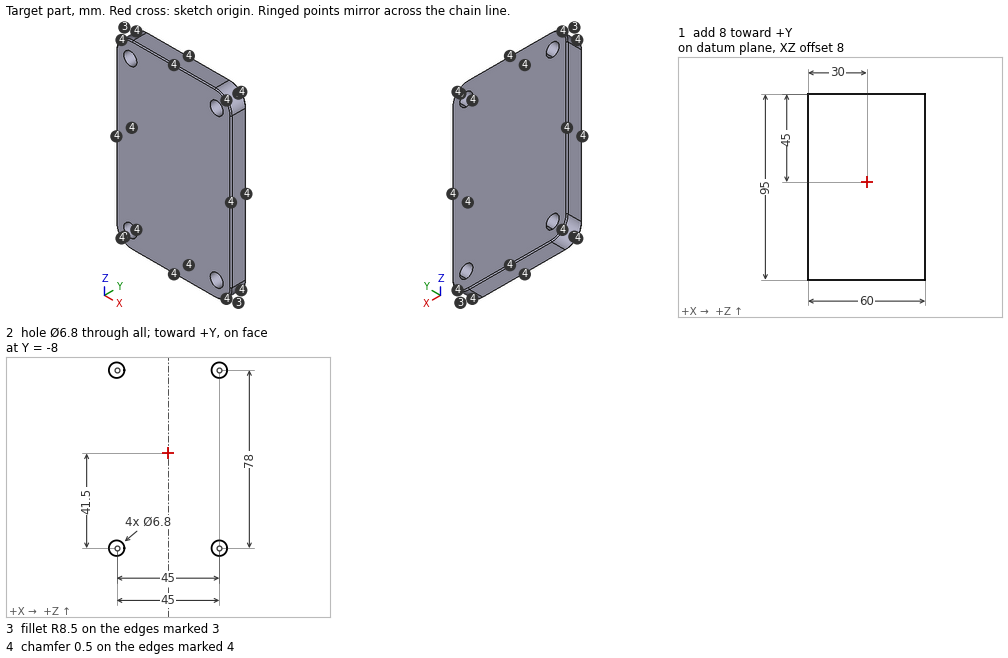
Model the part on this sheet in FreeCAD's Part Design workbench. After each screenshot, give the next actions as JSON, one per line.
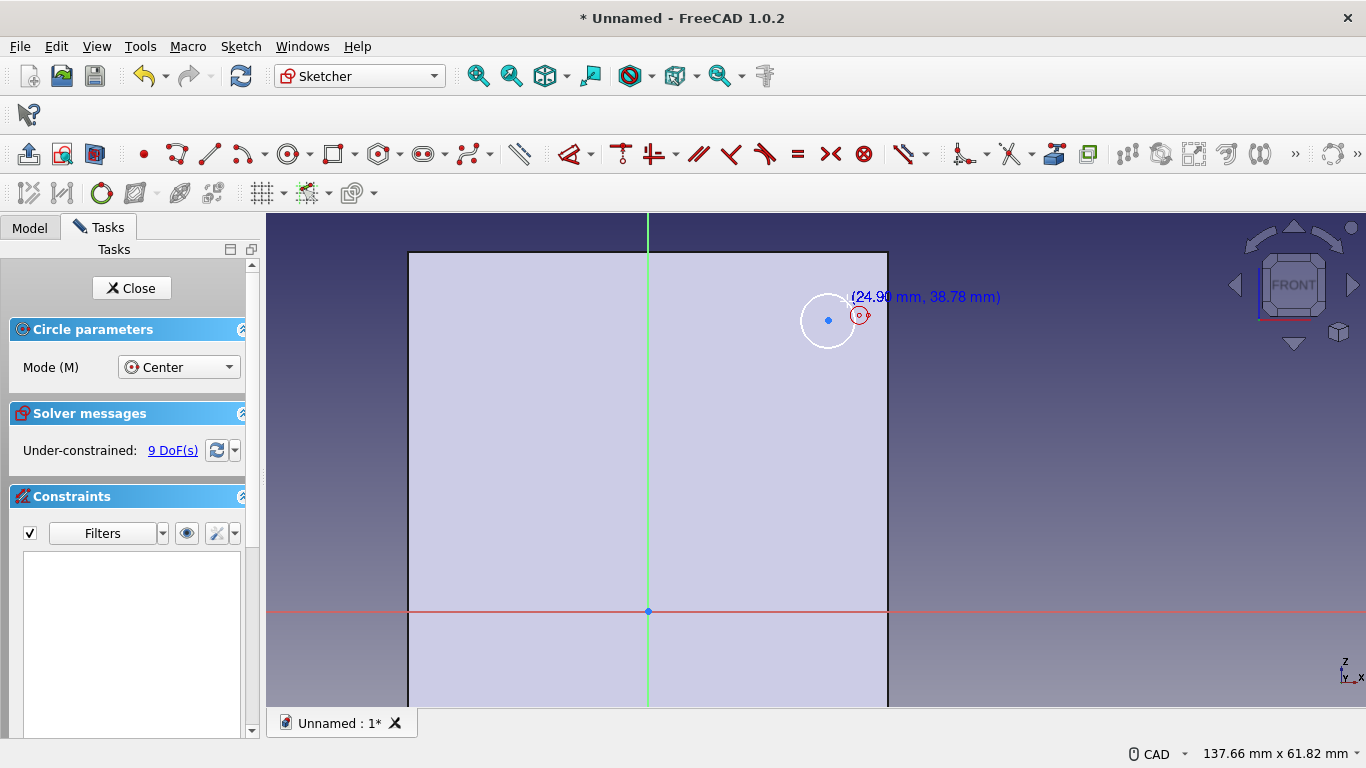
{"action": "left_click", "coordinate": [468, 320]}
{"action": "left_click", "coordinate": [487, 301]}
{"action": "key", "text": "Escape"}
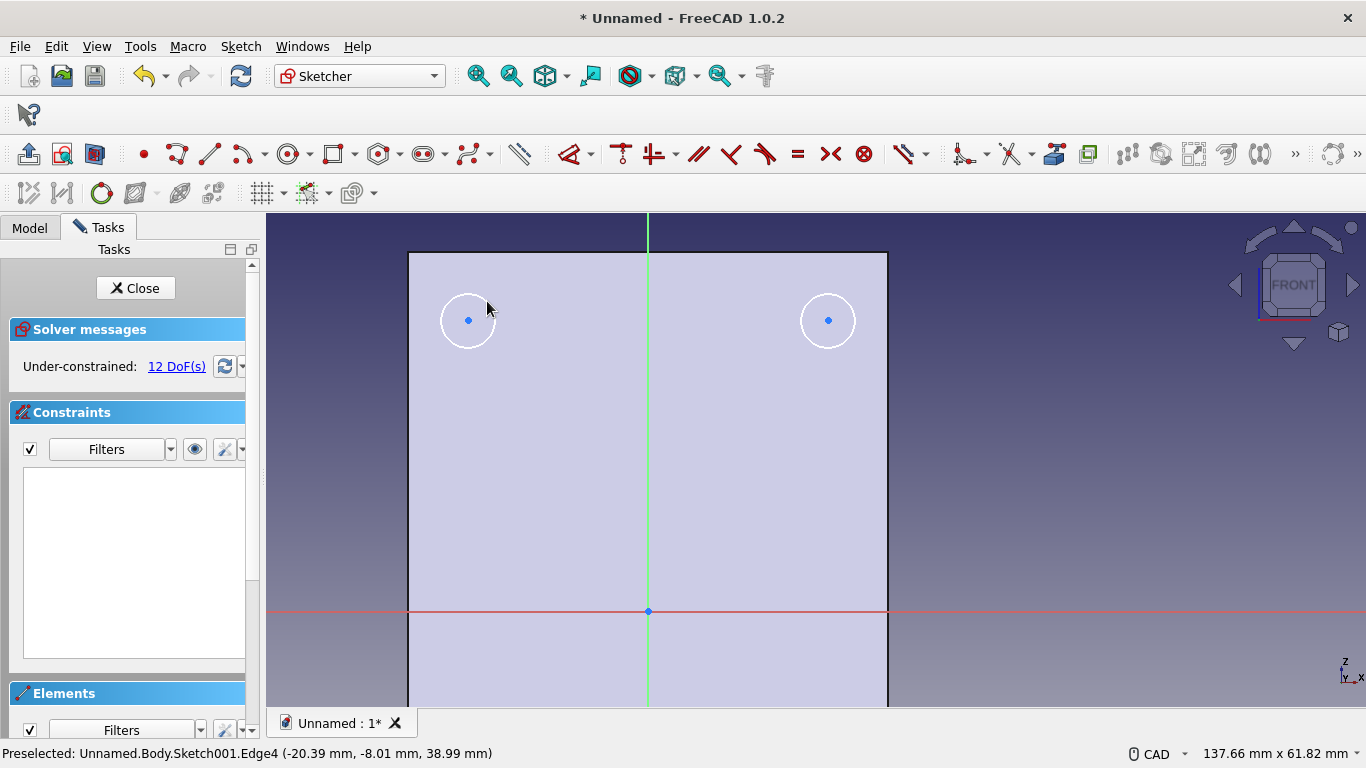
{"action": "scroll", "coordinate": [829, 320], "scroll_direction": "down", "scroll_amount": 4}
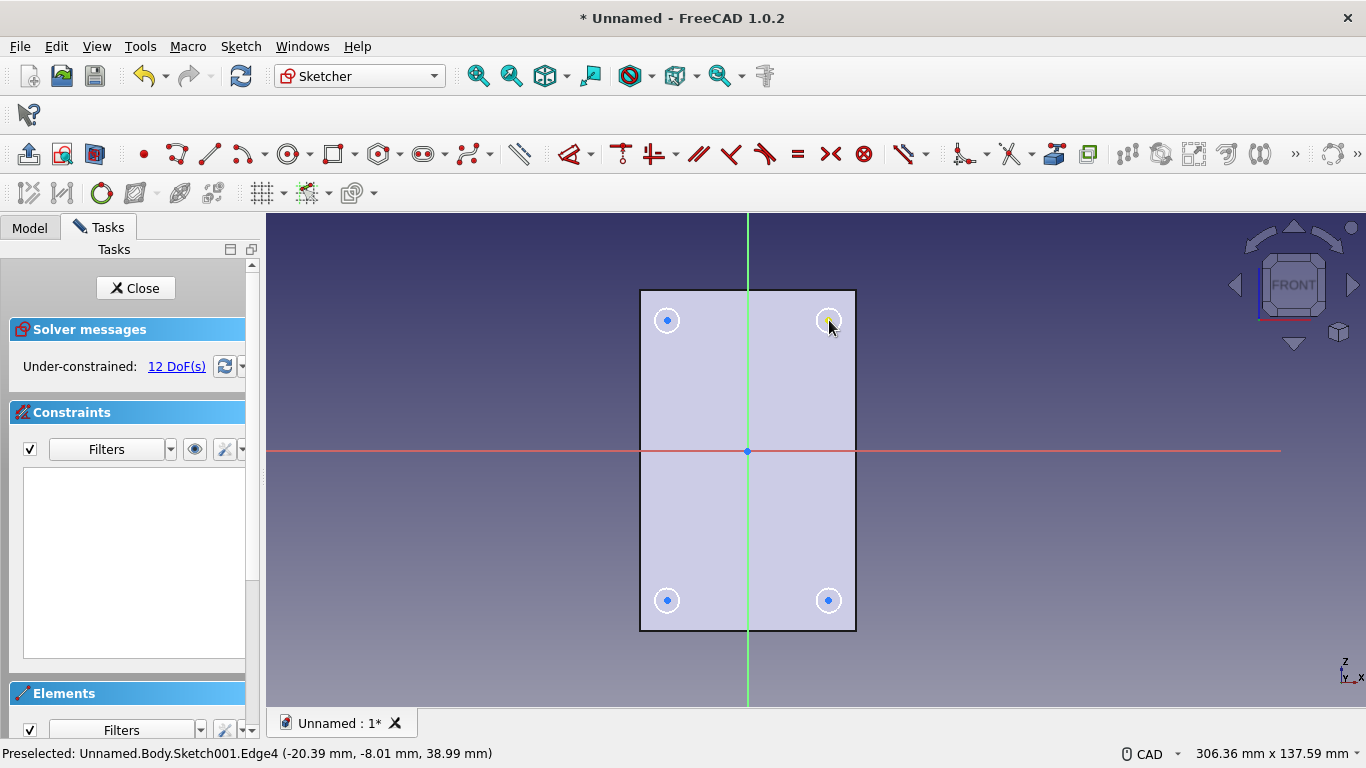
{"action": "left_click", "coordinate": [676, 592]}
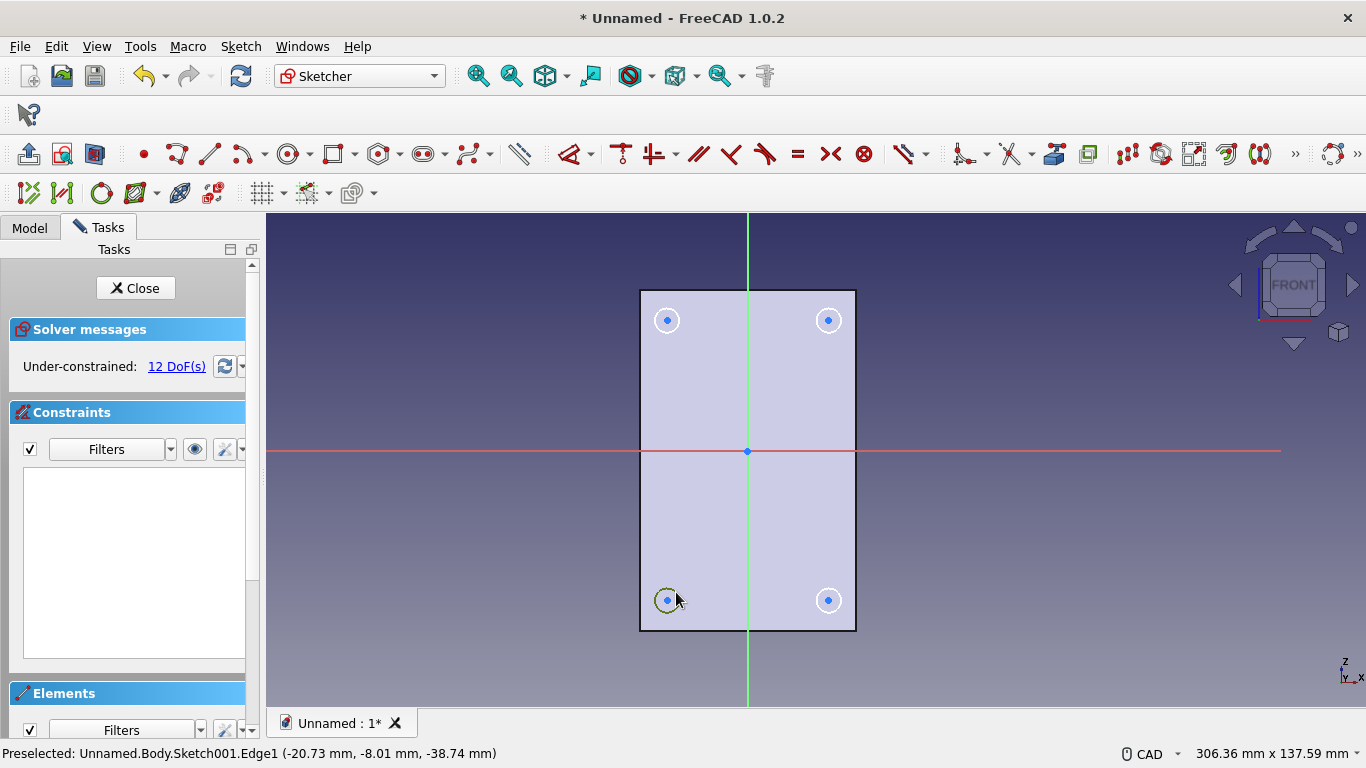
{"action": "left_click", "coordinate": [837, 592]}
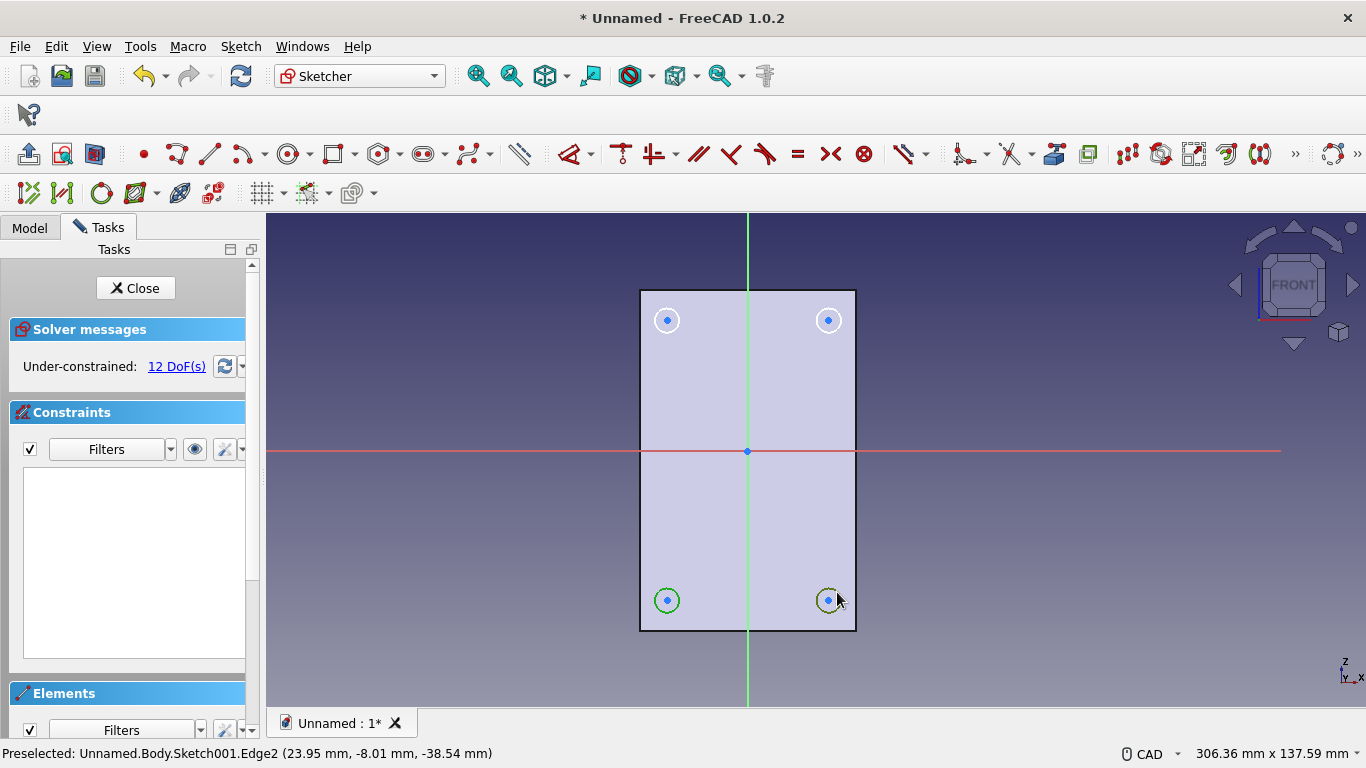
{"action": "left_click", "coordinate": [837, 312]}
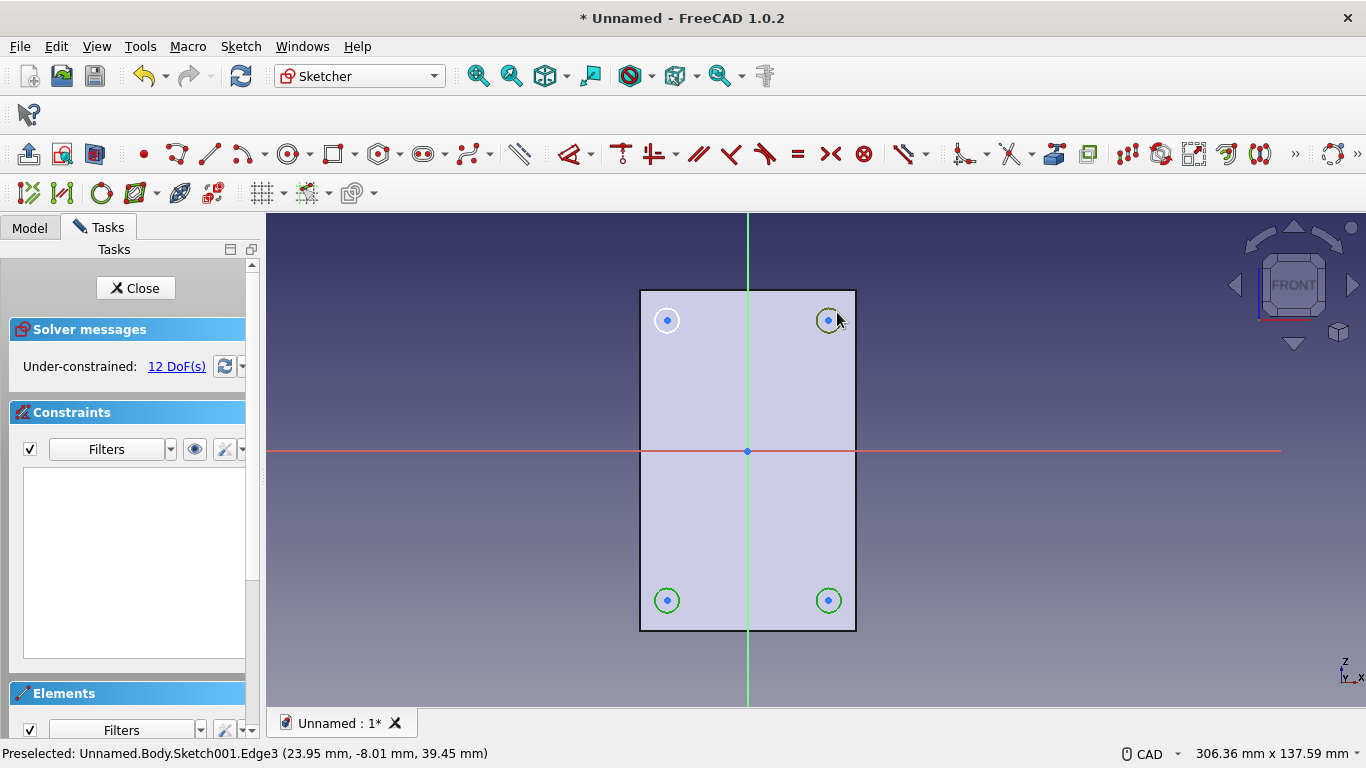
{"action": "left_click", "coordinate": [676, 312]}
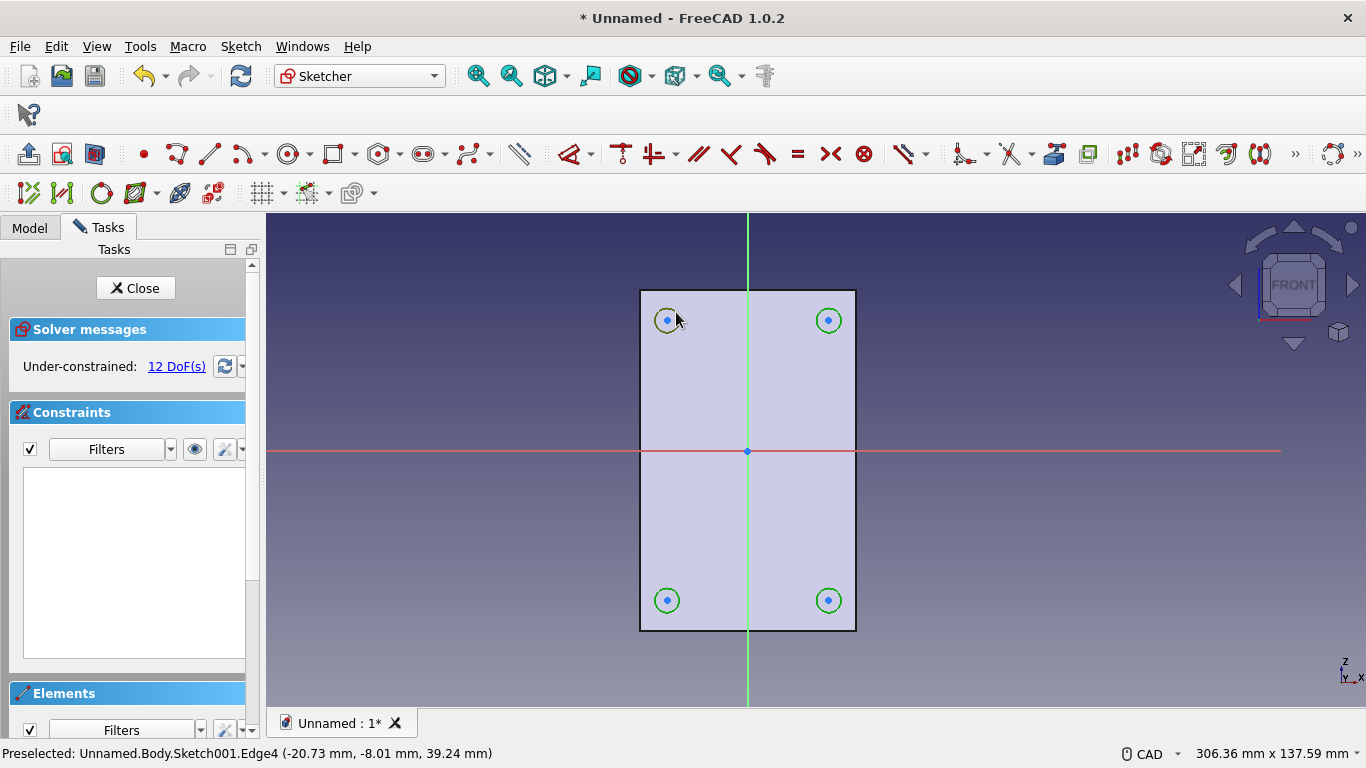
{"action": "left_click", "coordinate": [798, 154]}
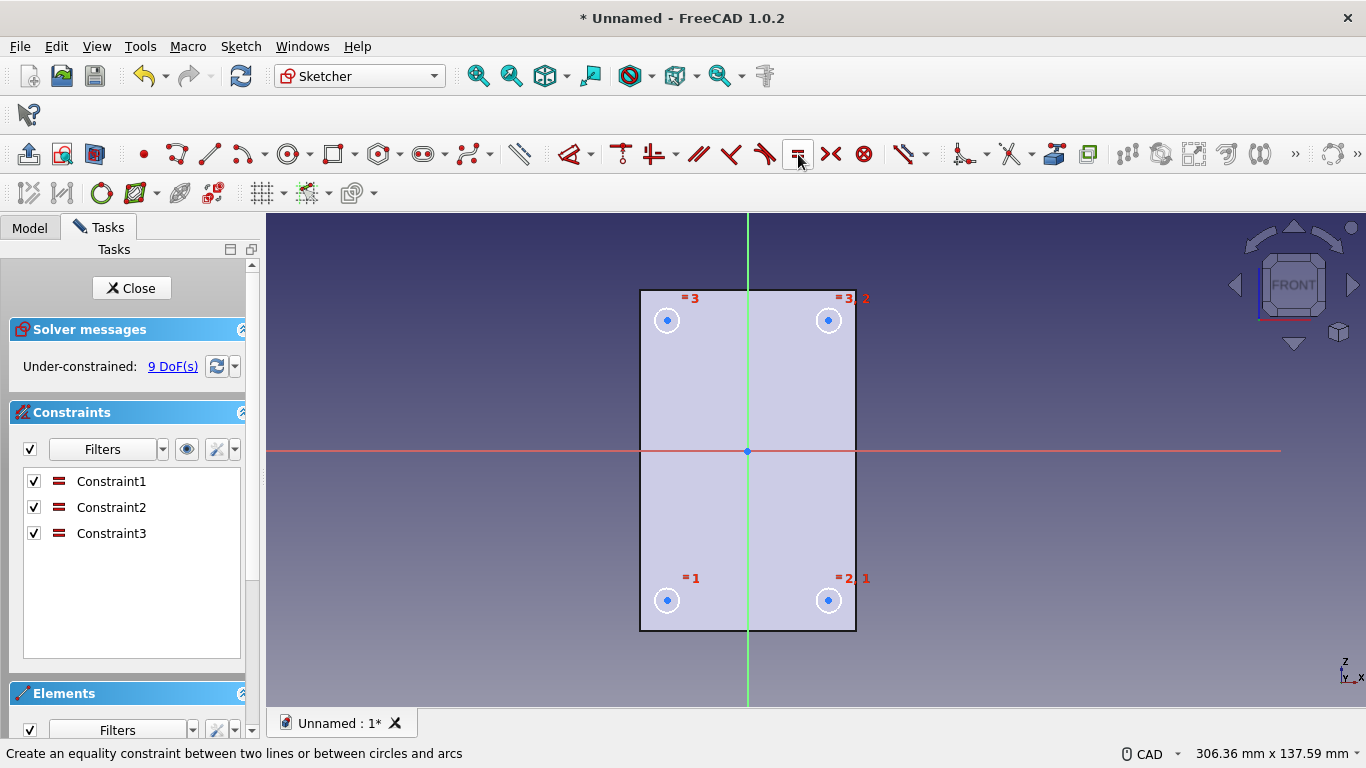
{"action": "left_click", "coordinate": [667, 601]}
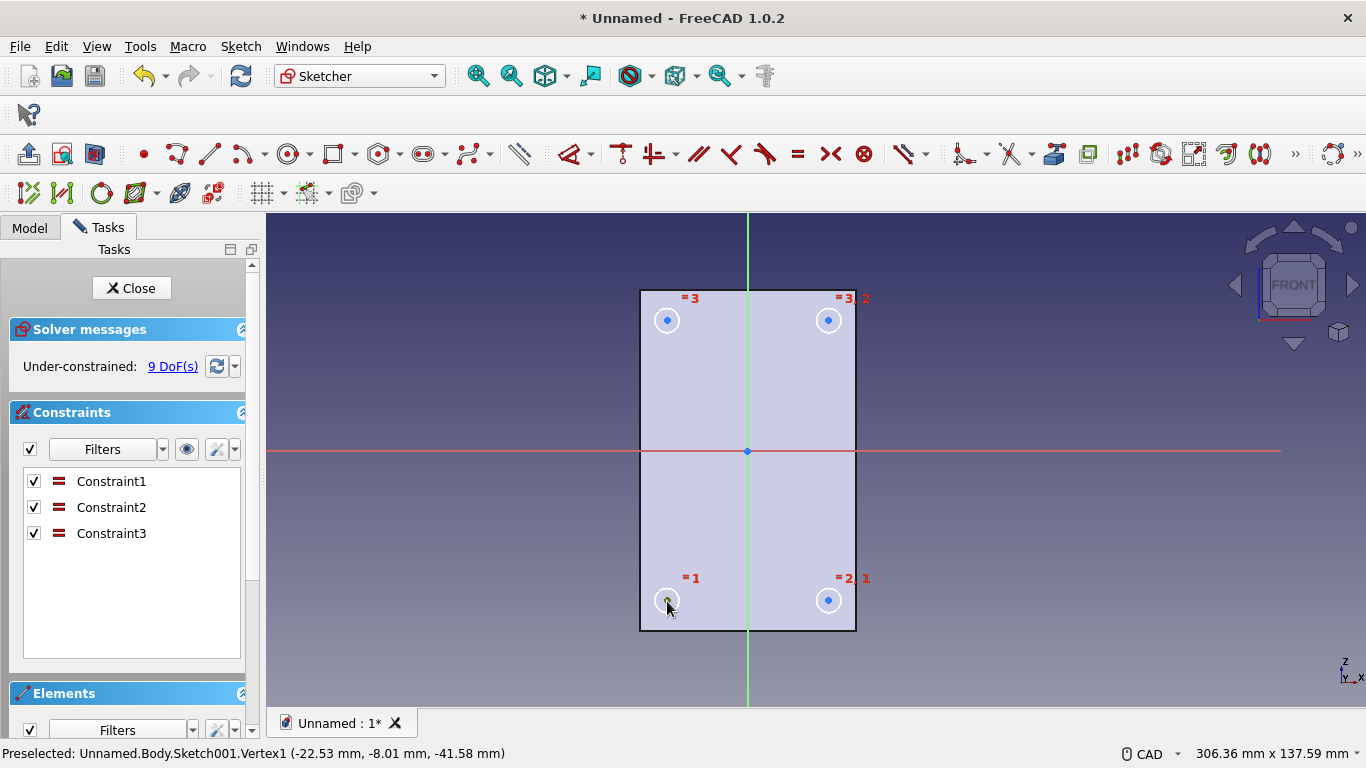
{"action": "left_click", "coordinate": [829, 601]}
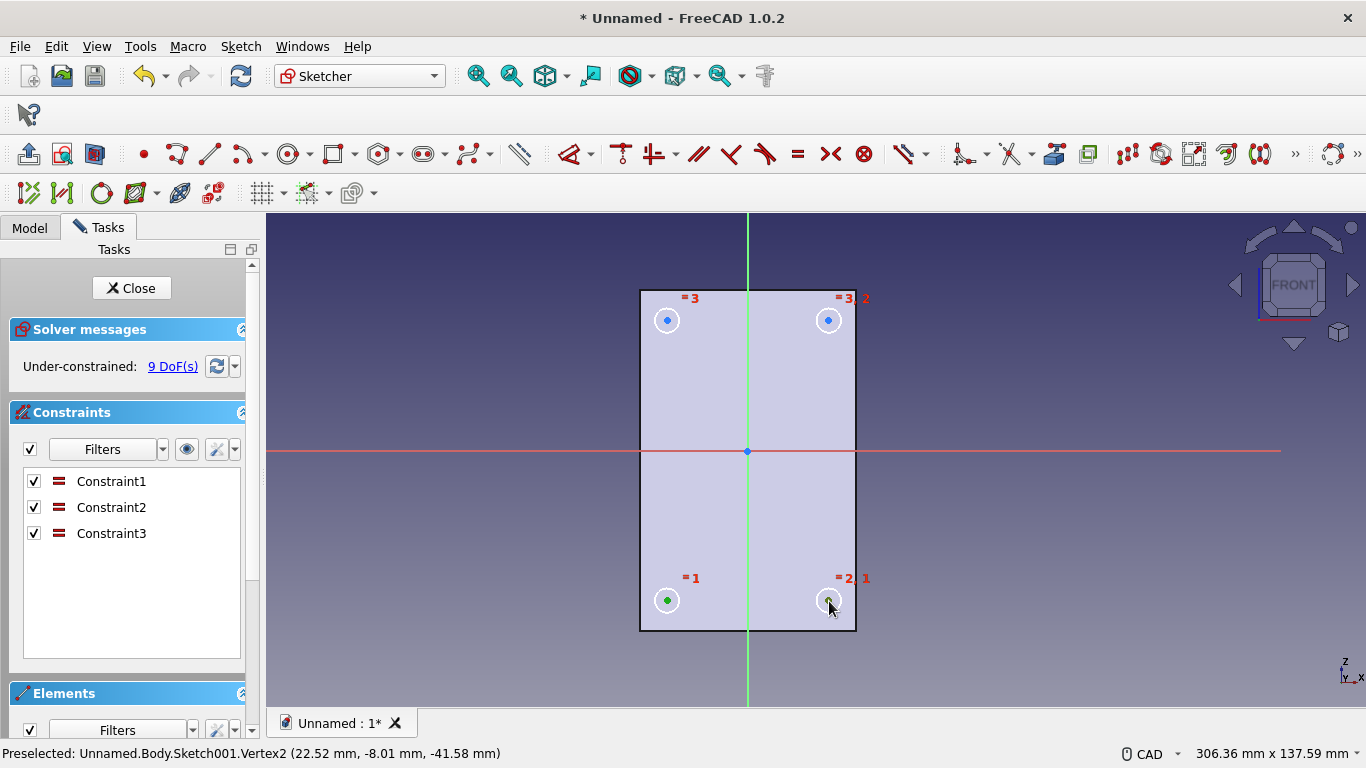
{"action": "left_click", "coordinate": [748, 648]}